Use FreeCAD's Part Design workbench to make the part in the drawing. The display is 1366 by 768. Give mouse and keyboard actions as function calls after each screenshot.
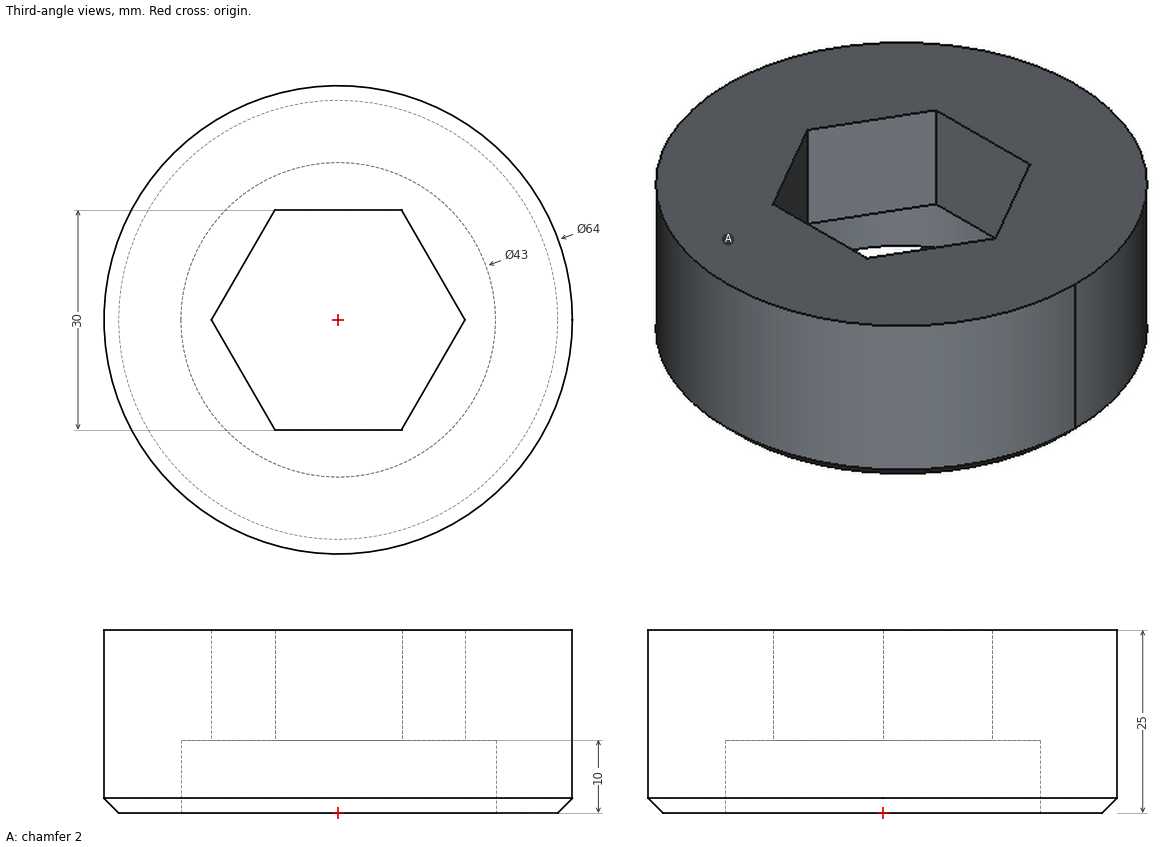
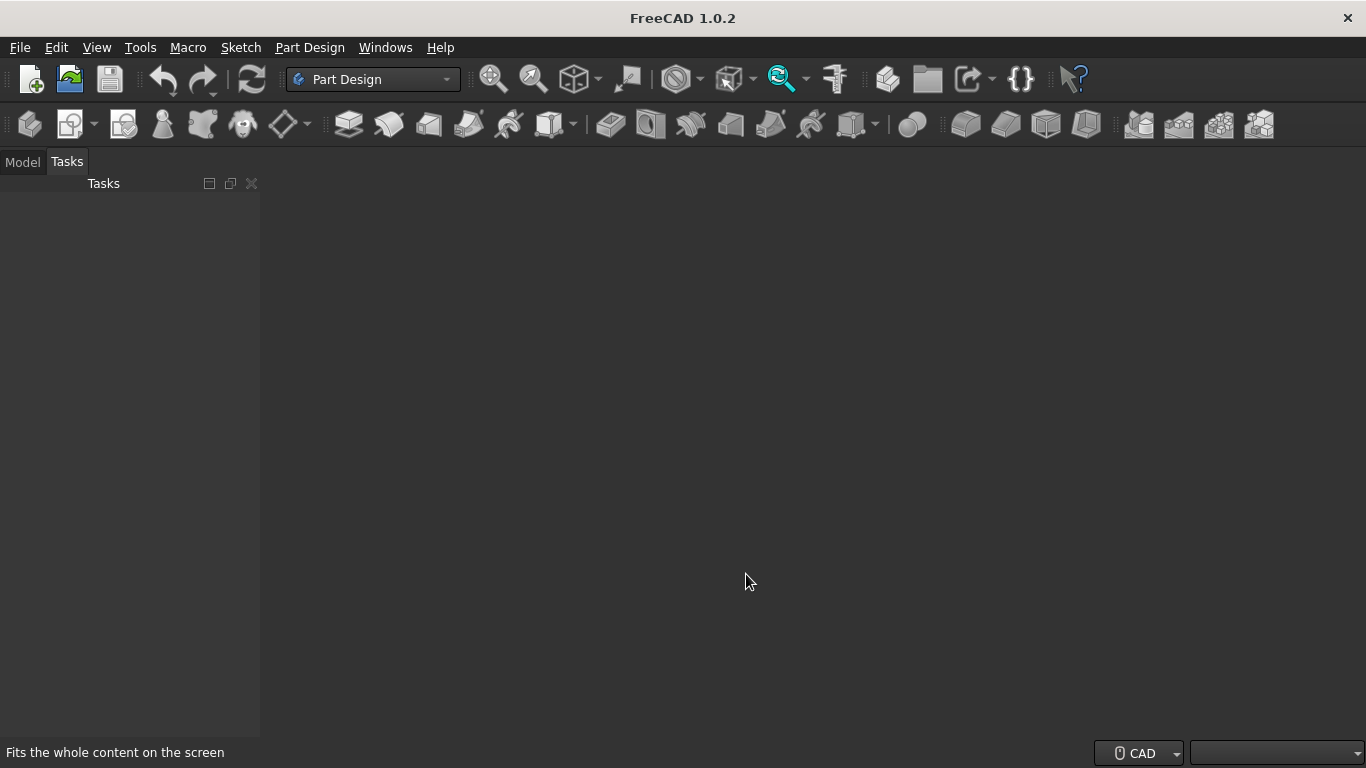
key(ctrl+n)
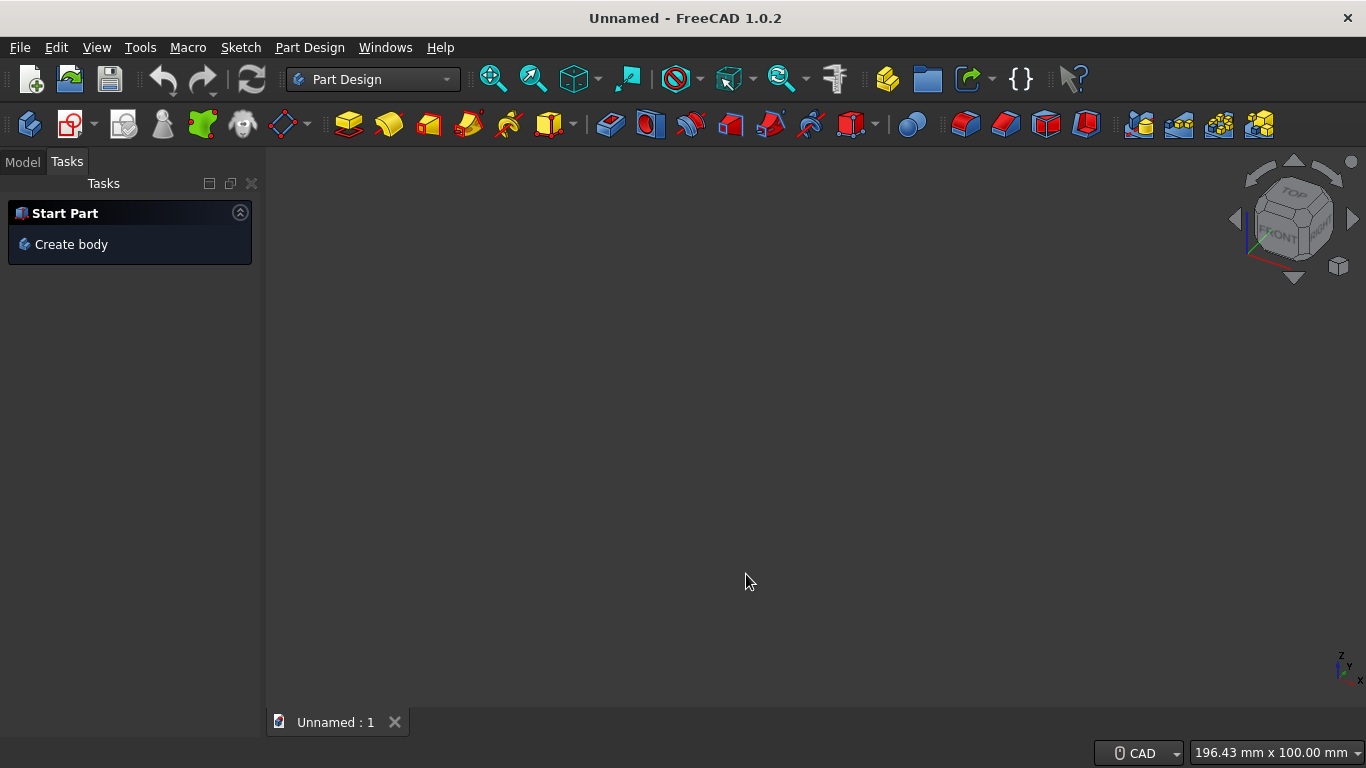
click(70, 124)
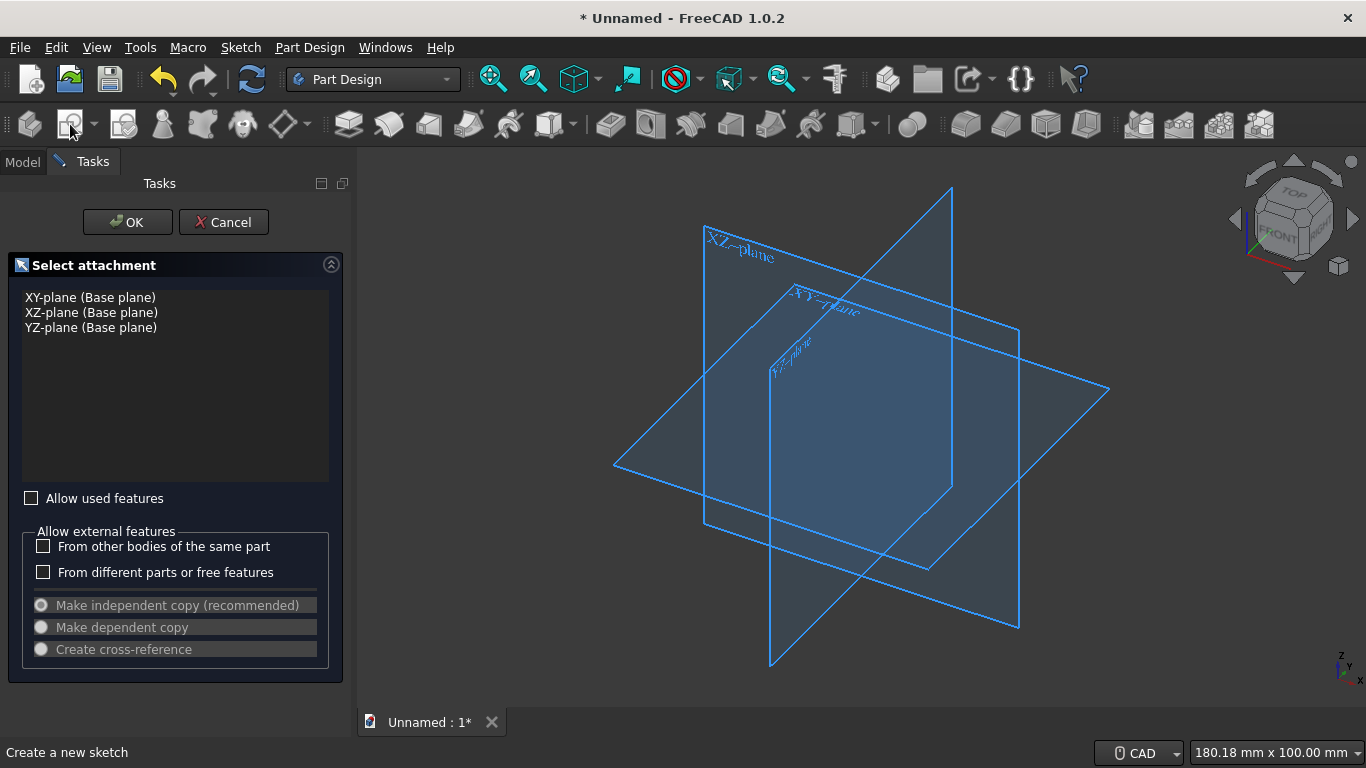
click(82, 298)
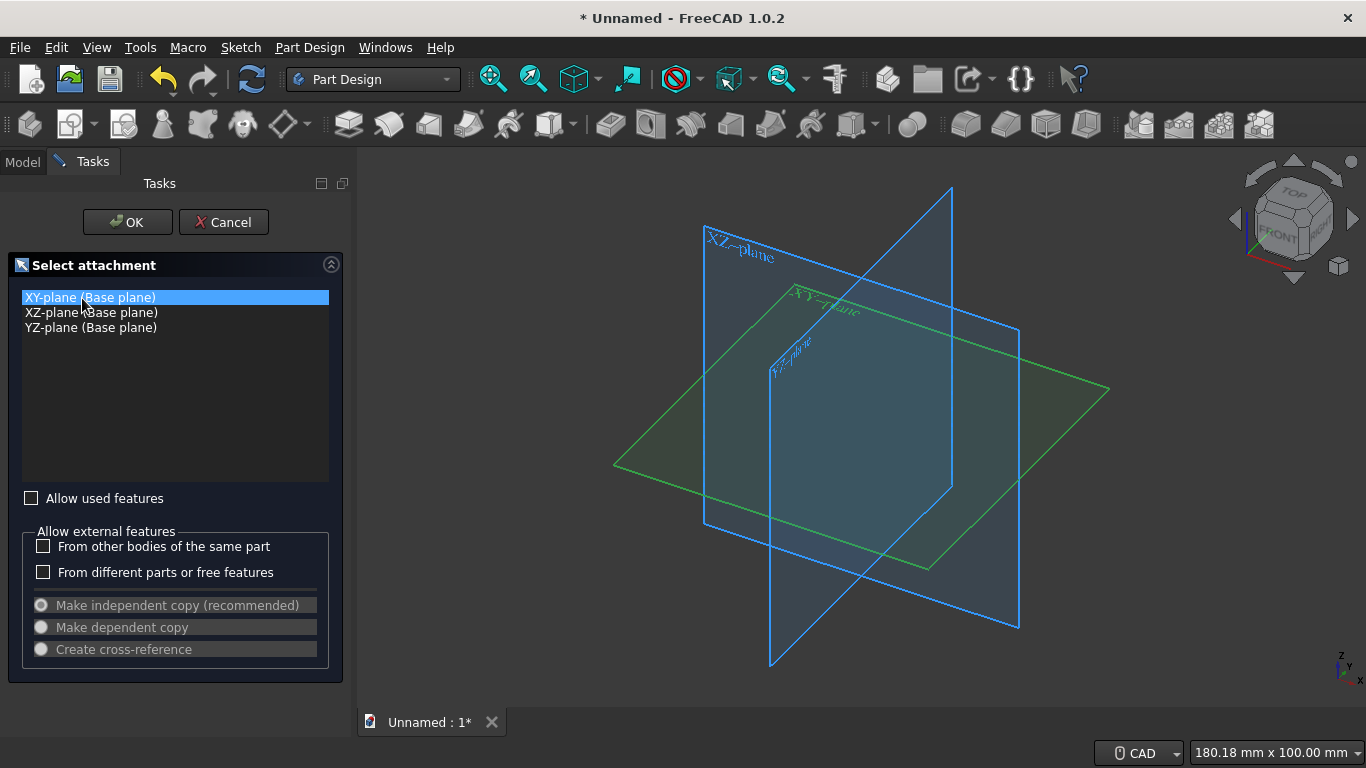
click(128, 222)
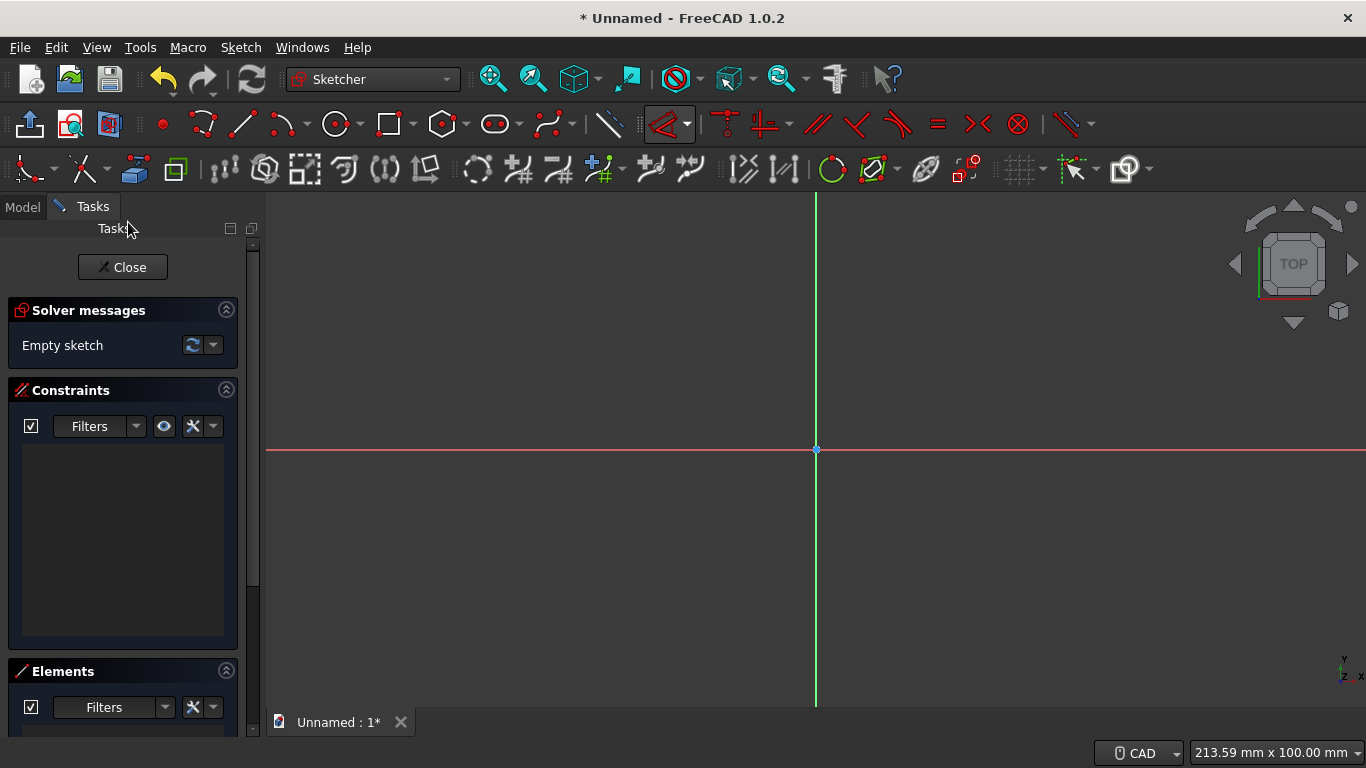
click(336, 124)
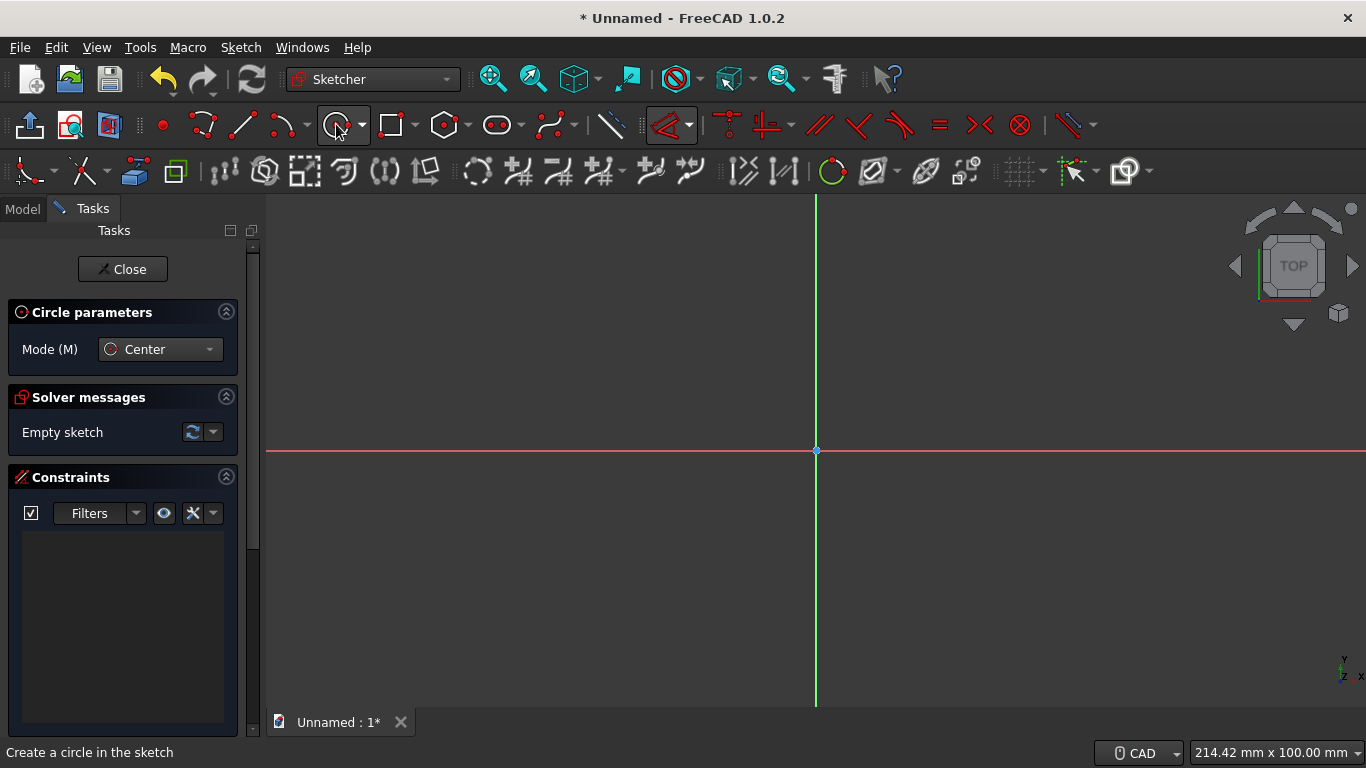
click(816, 450)
click(932, 334)
key(Escape)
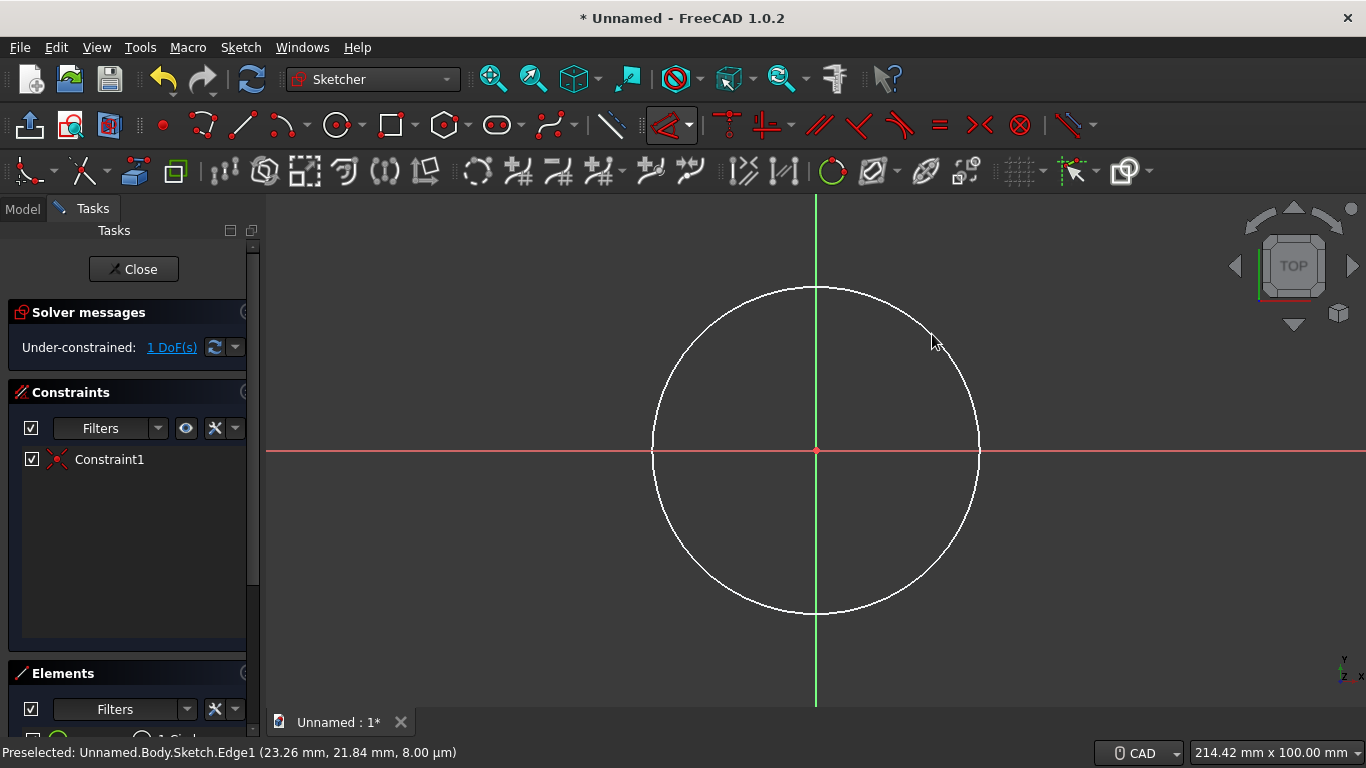
key(d)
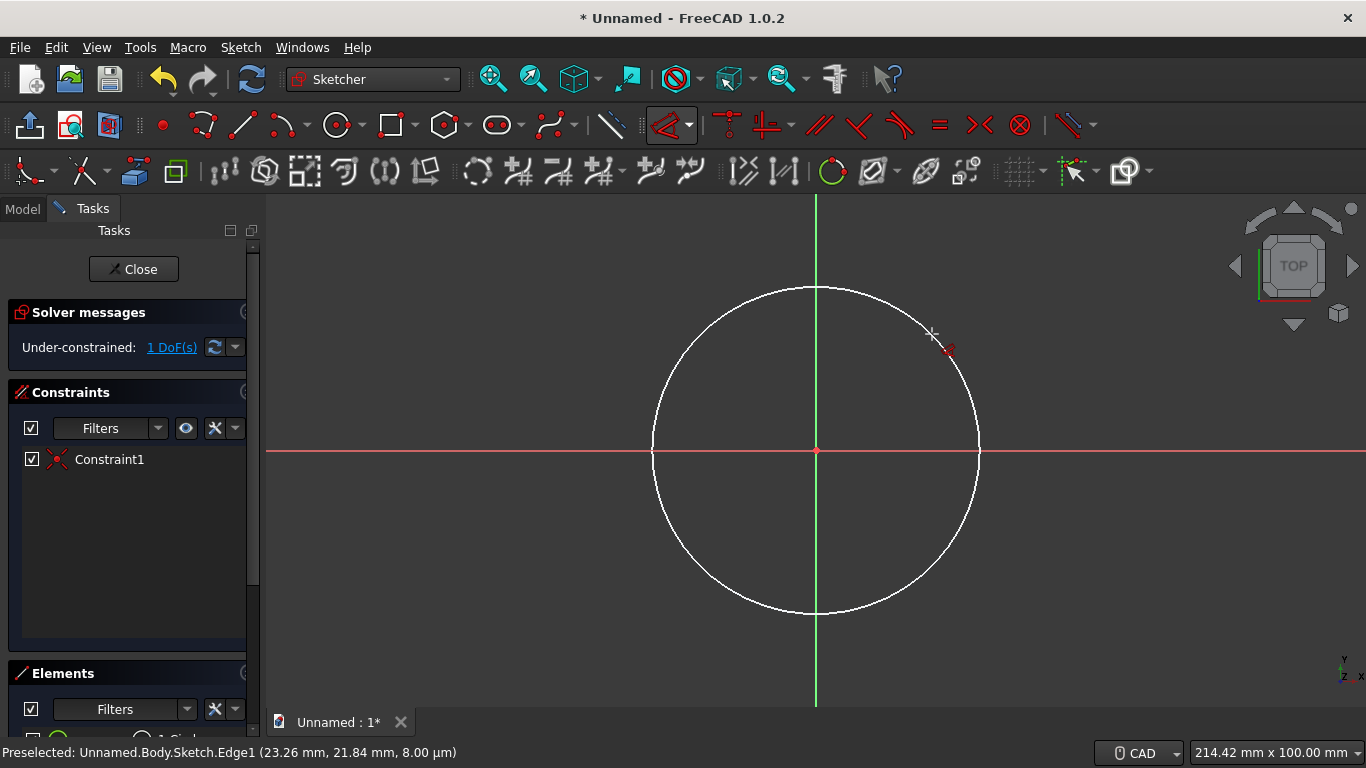
click(931, 334)
click(953, 311)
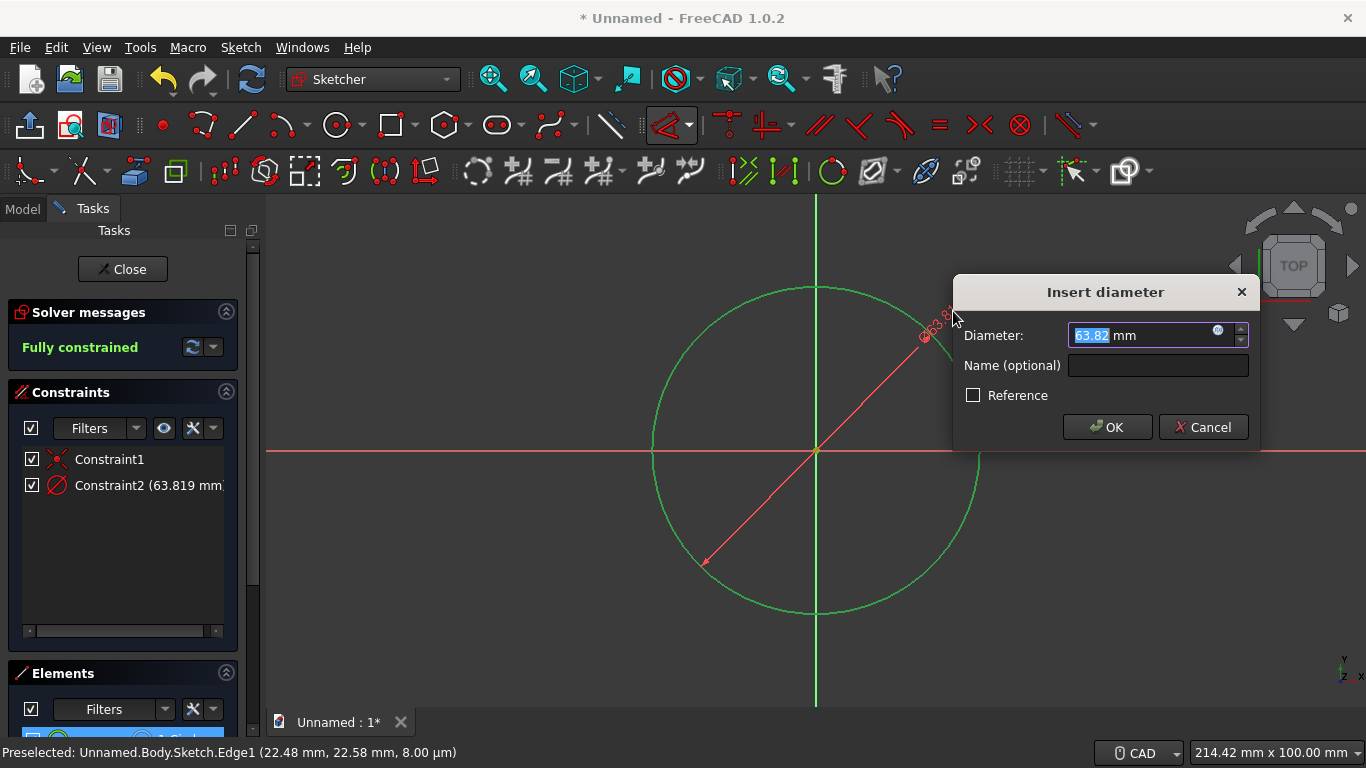
text(64)
key(Return)
key(Escape)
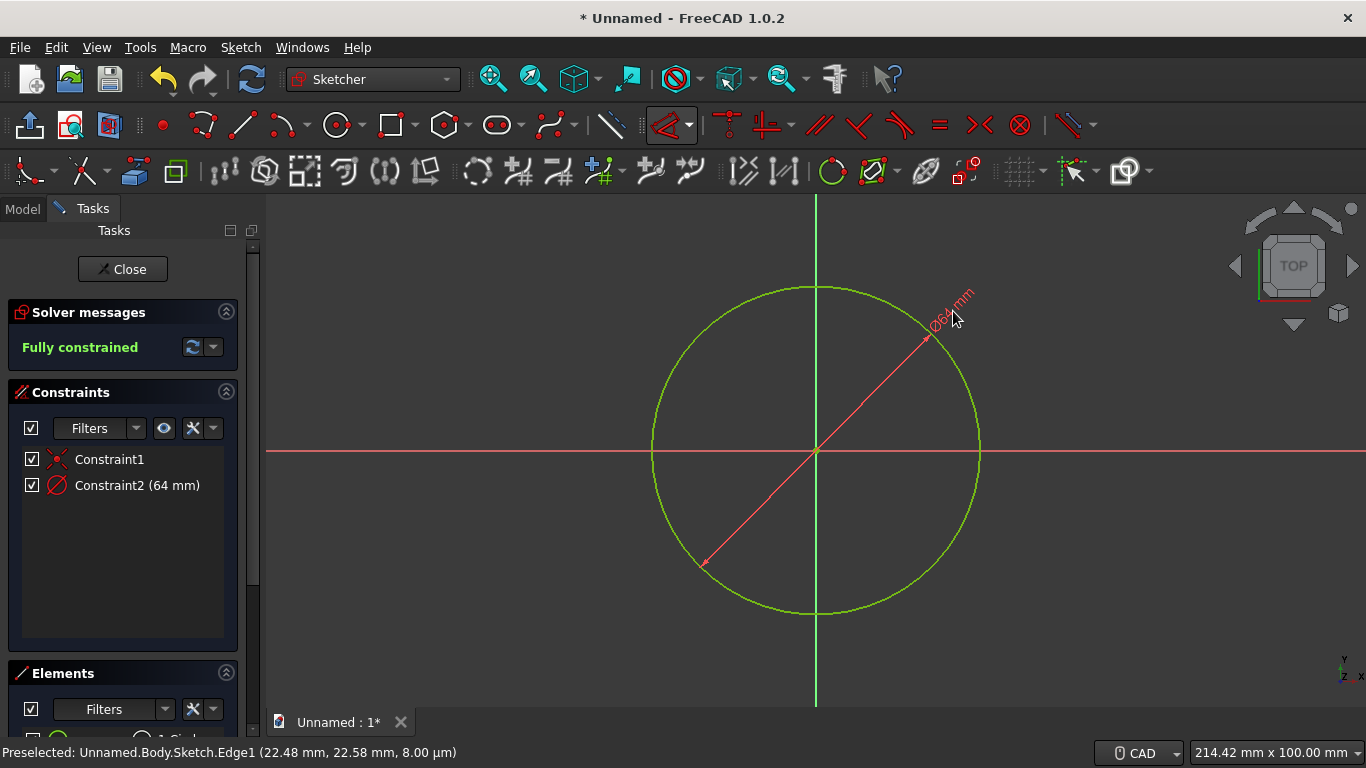
click(123, 269)